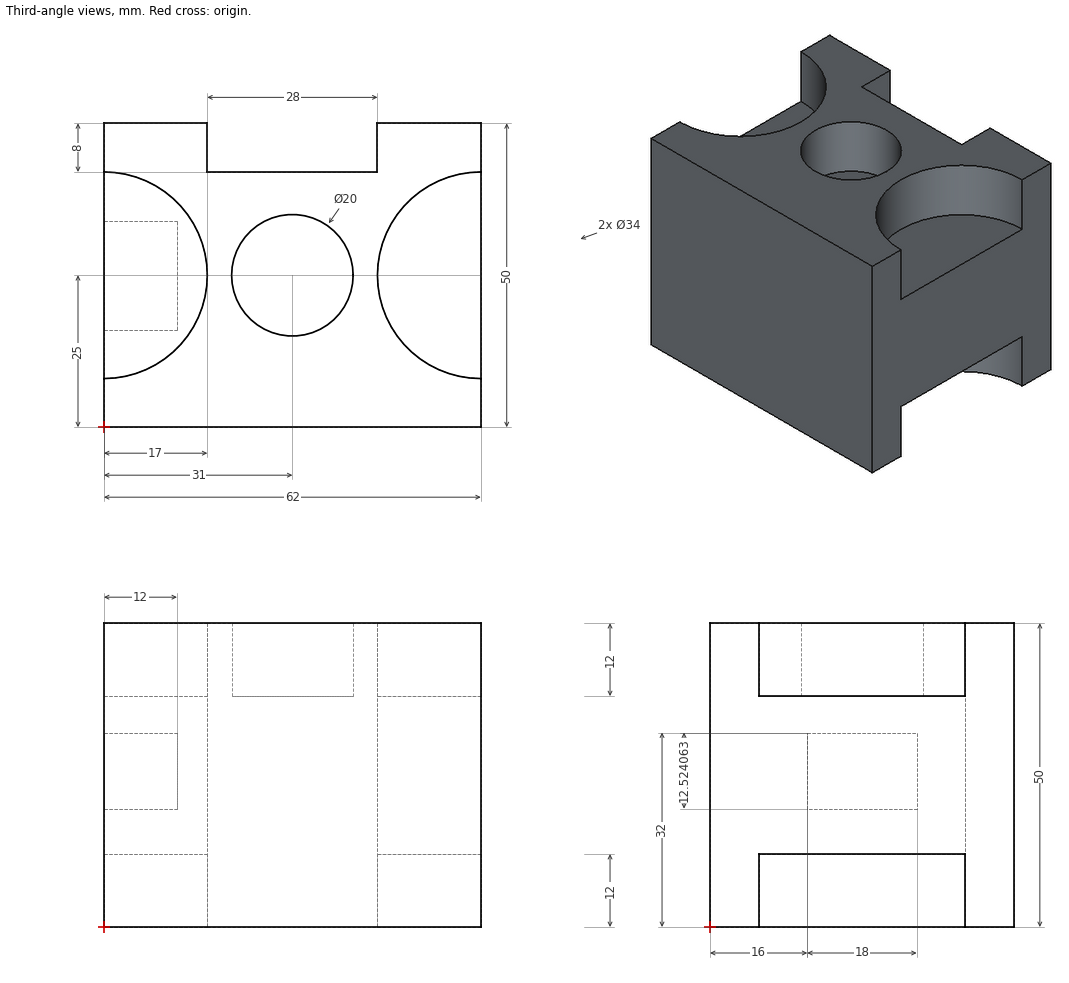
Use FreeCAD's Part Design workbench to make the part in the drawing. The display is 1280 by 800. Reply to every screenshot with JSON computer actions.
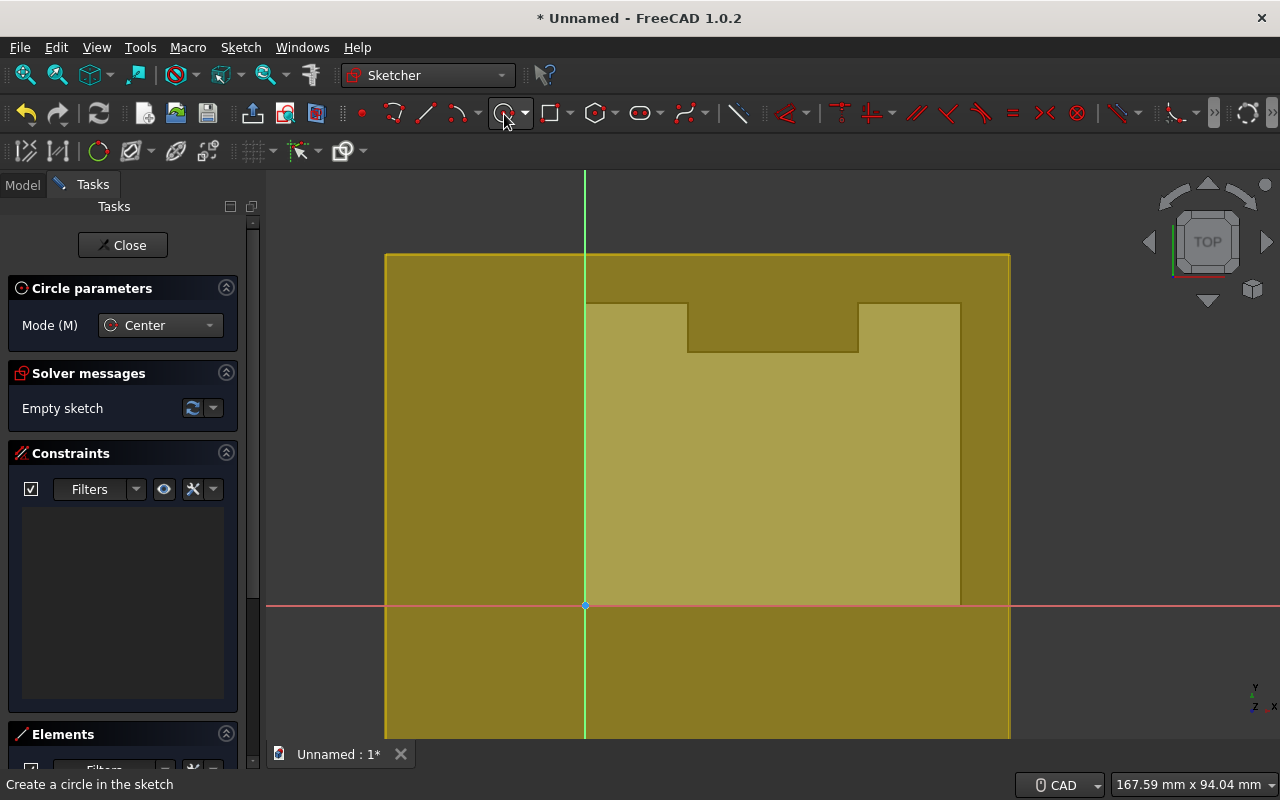
{"action": "left_click", "coordinate": [961, 455]}
{"action": "left_click", "coordinate": [1033, 382]}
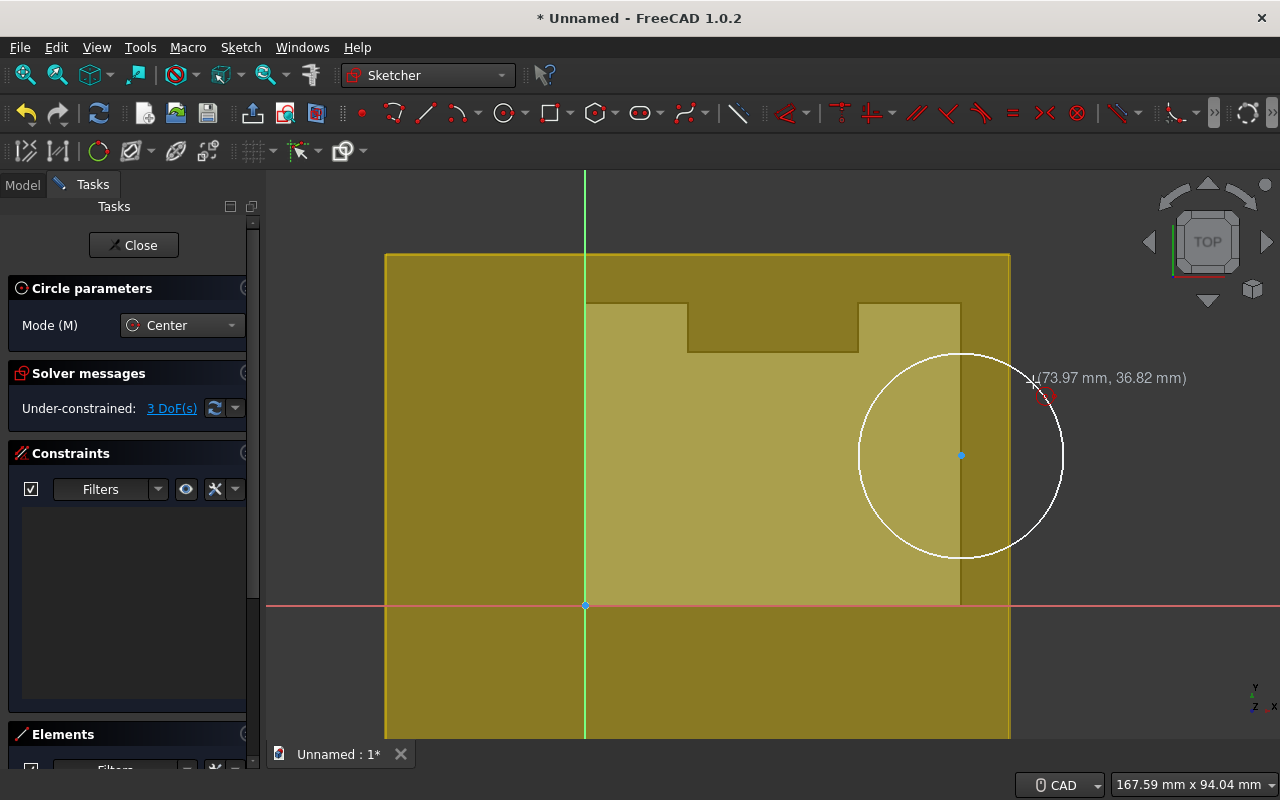
{"action": "left_click", "coordinate": [585, 455]}
{"action": "left_click", "coordinate": [658, 382]}
{"action": "key", "text": "Escape"}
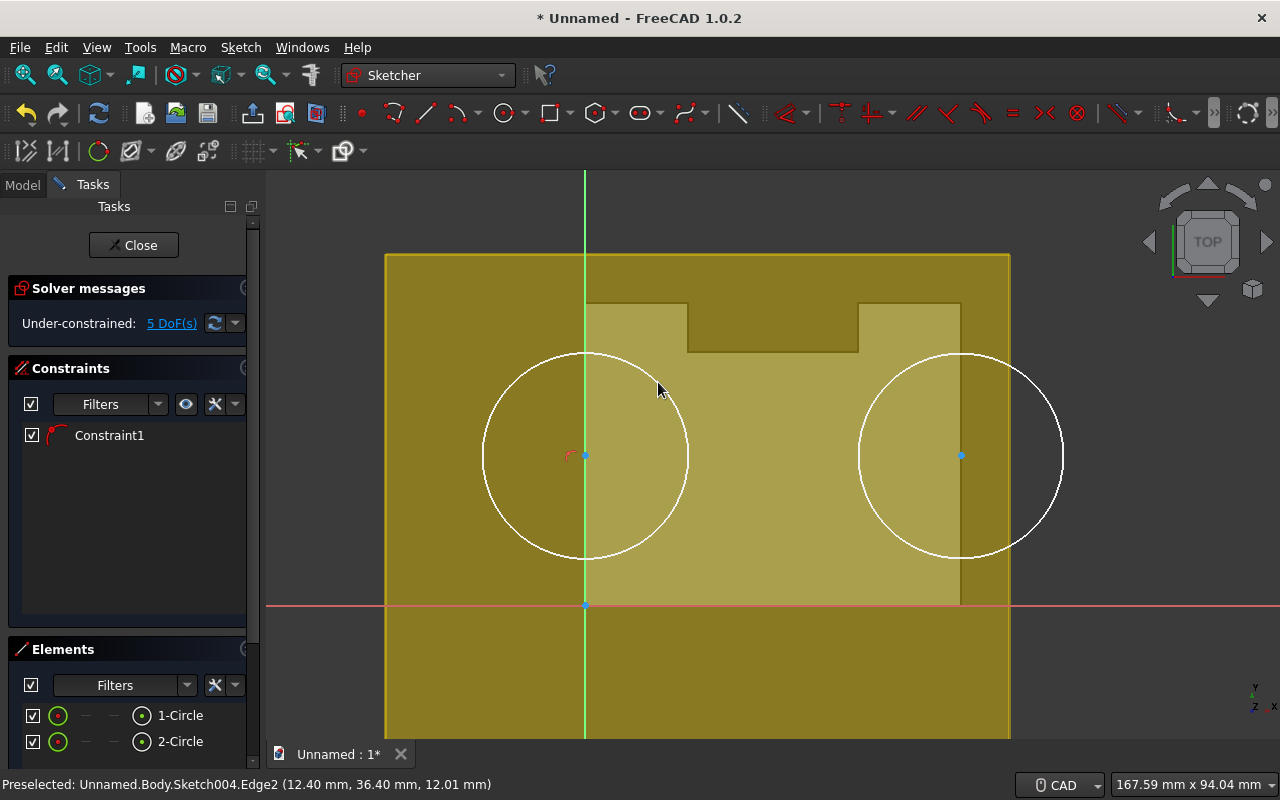
{"action": "left_click", "coordinate": [1033, 383]}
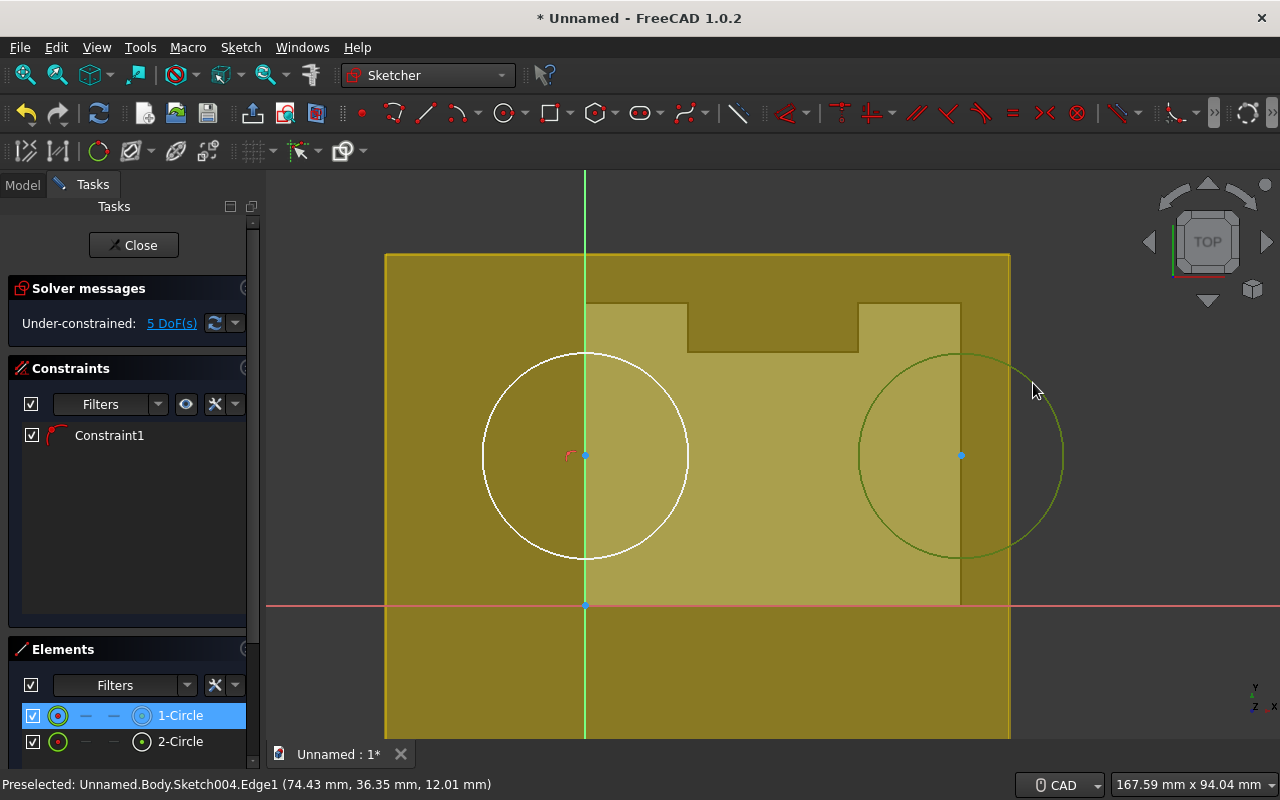
{"action": "left_click", "coordinate": [658, 383]}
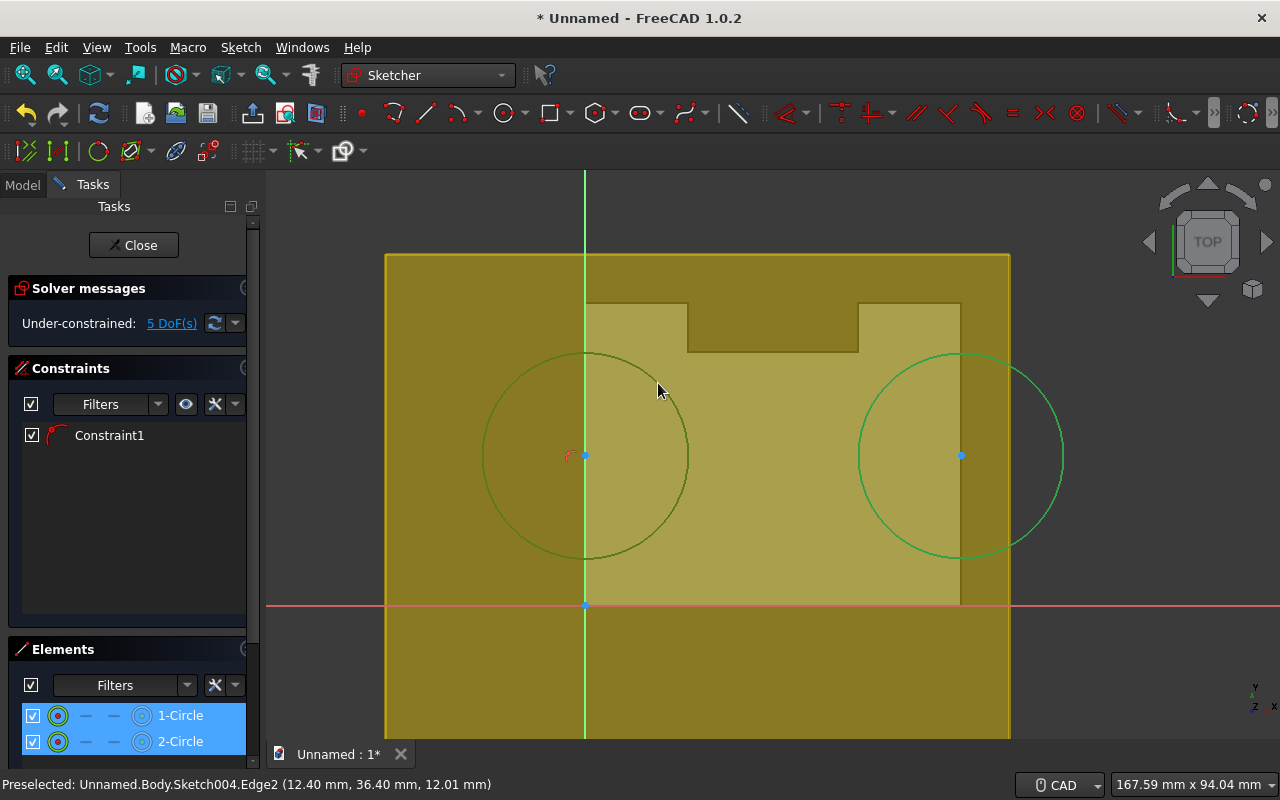
{"action": "left_click", "coordinate": [1014, 114]}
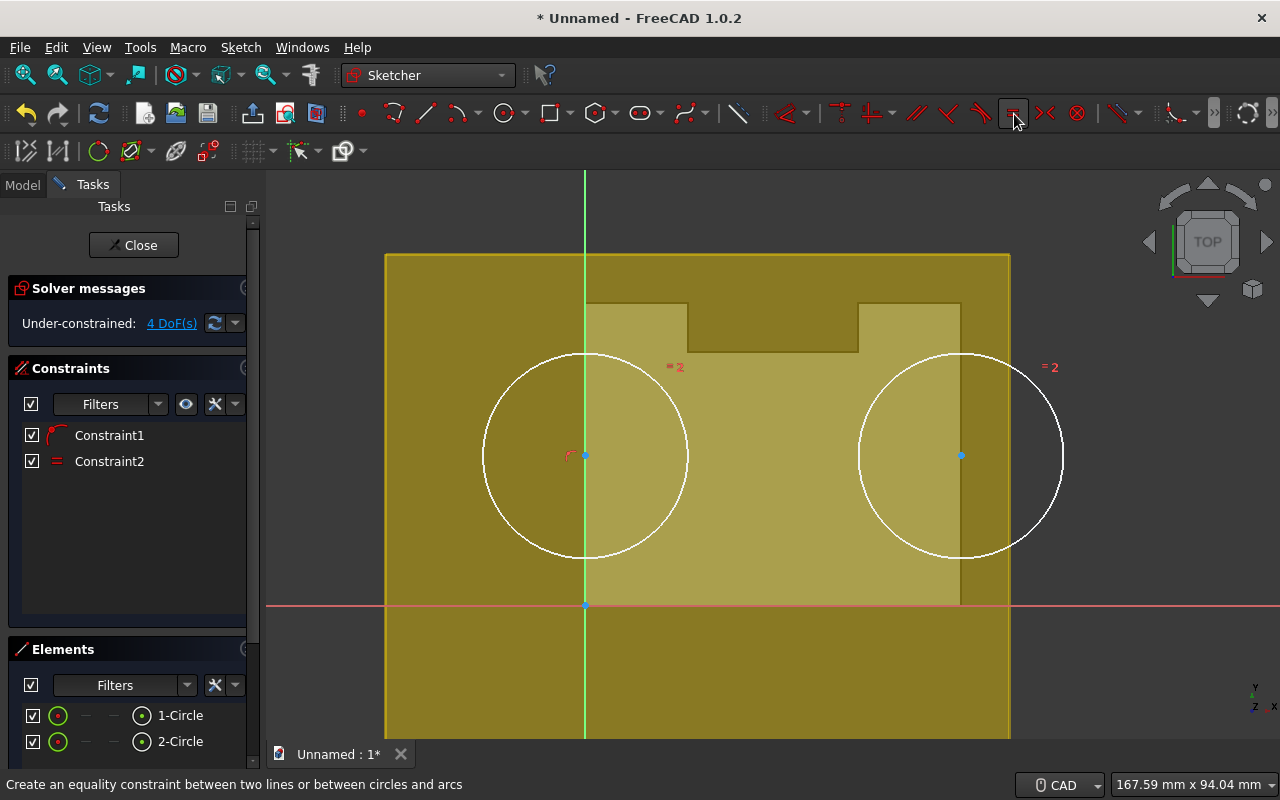
{"action": "left_click", "coordinate": [961, 456]}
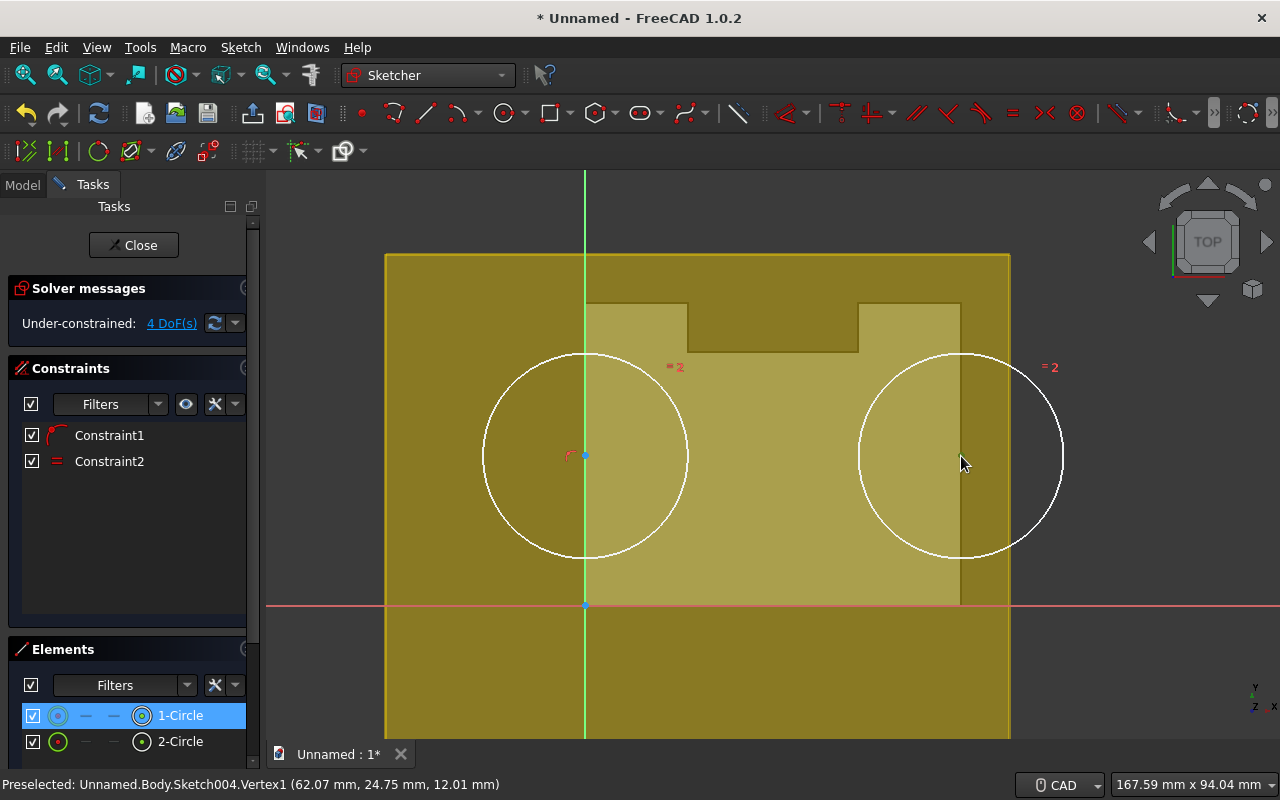
{"action": "left_click", "coordinate": [585, 456]}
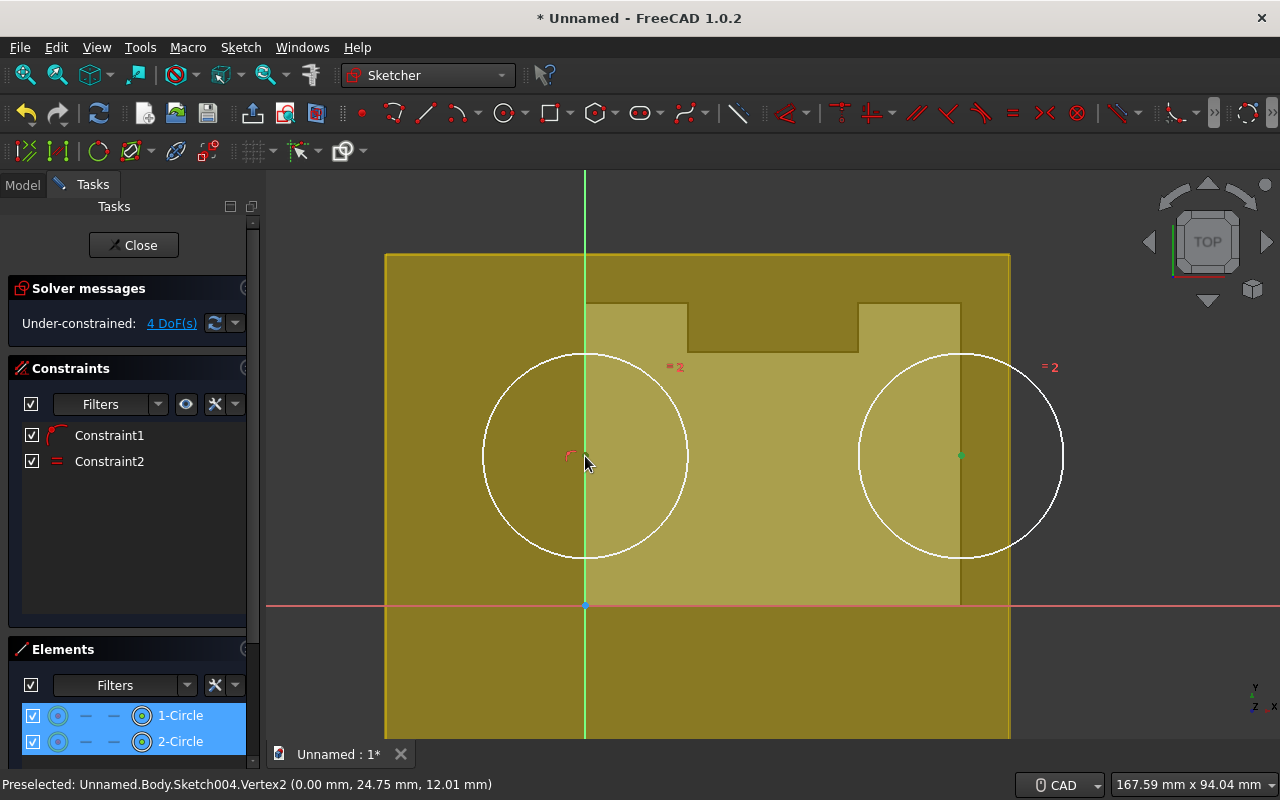
{"action": "key", "text": "h"}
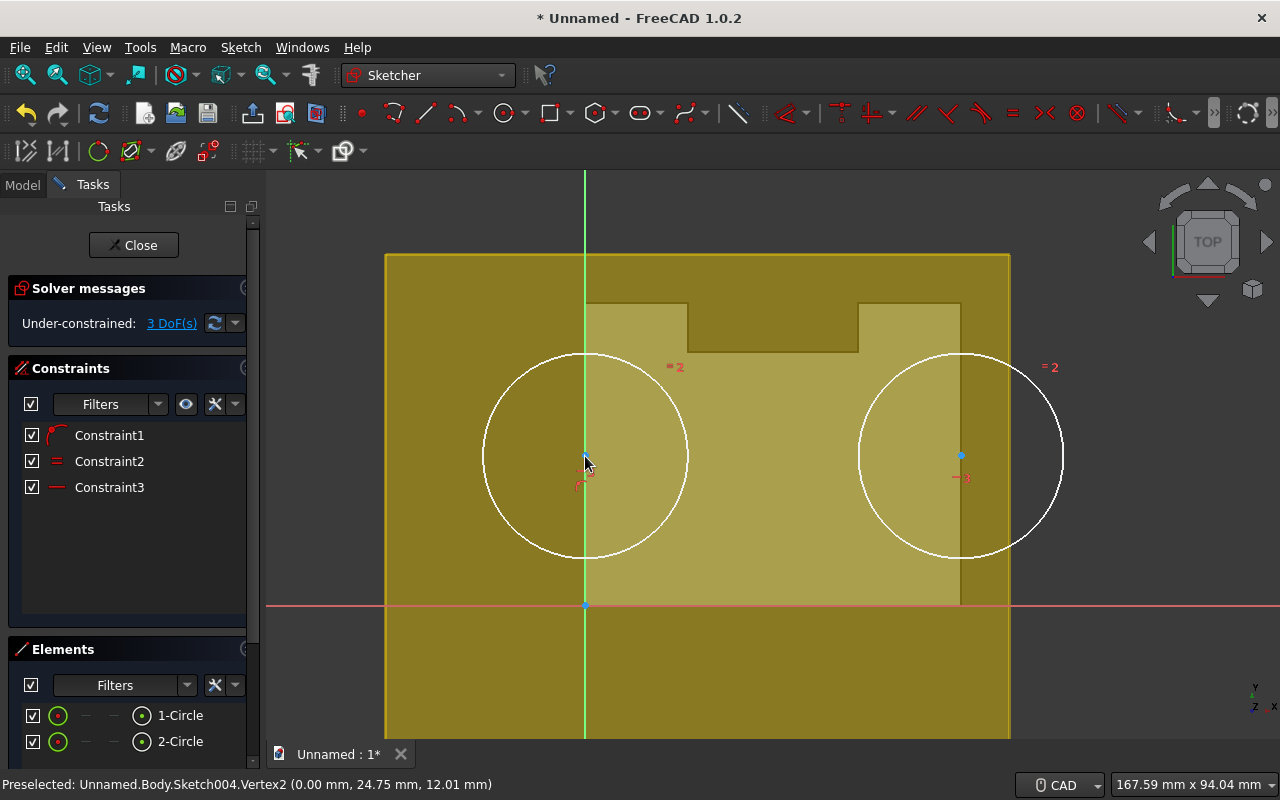
{"action": "left_click", "coordinate": [786, 114]}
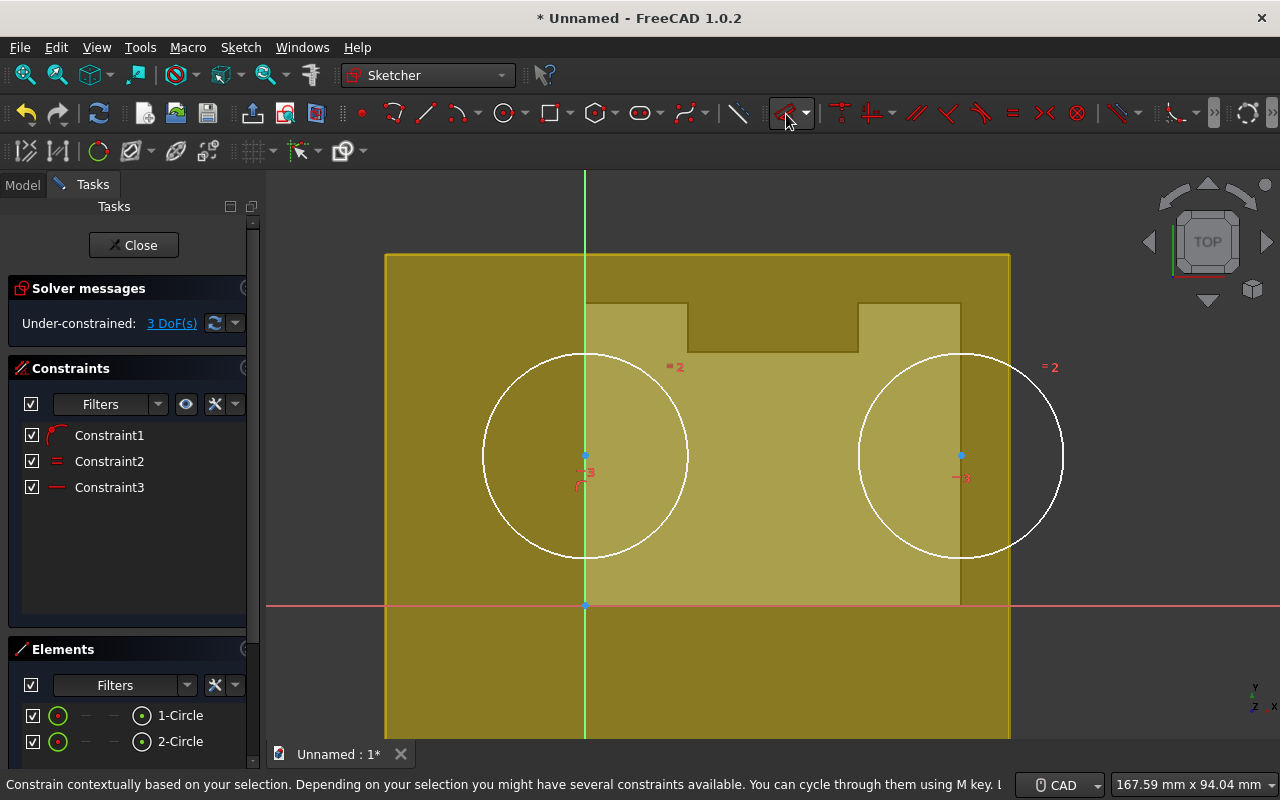
{"action": "left_click", "coordinate": [1033, 383]}
{"action": "left_click", "coordinate": [1055, 360]}